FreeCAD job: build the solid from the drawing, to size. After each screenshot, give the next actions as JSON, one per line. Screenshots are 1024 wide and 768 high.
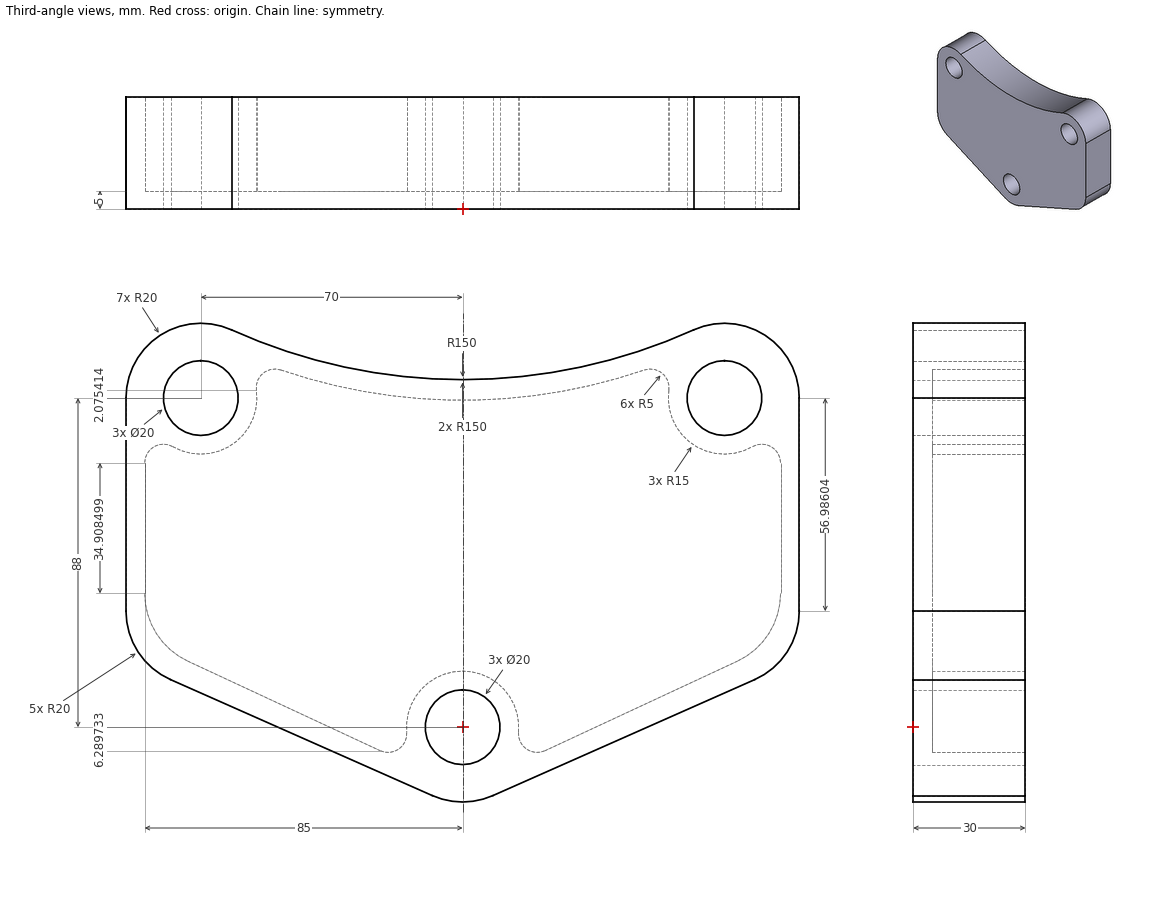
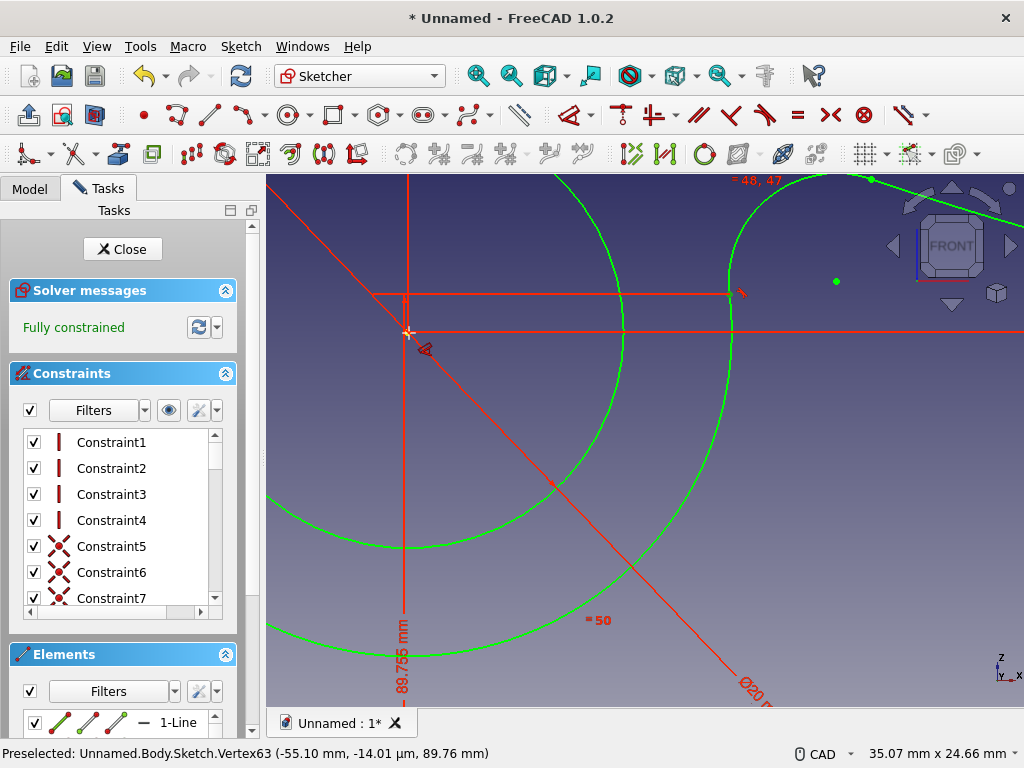
{"action": "left_click", "coordinate": [408, 332]}
{"action": "left_click", "coordinate": [374, 313]}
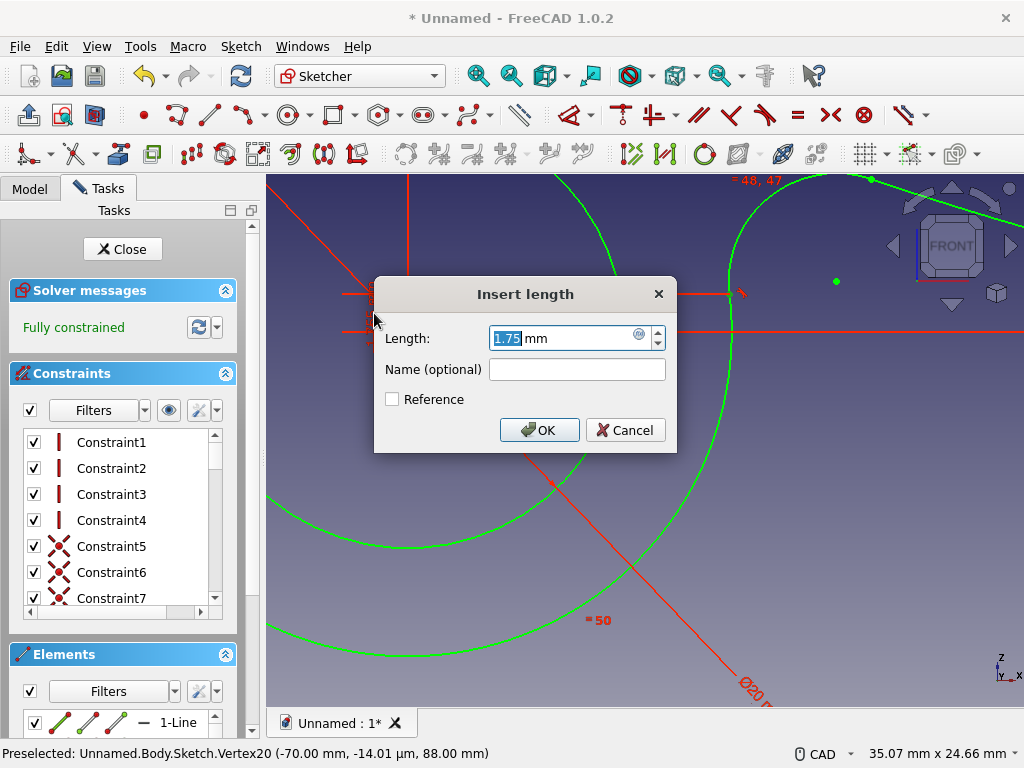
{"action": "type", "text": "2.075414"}
{"action": "key", "text": "Return"}
{"action": "key", "text": "Escape"}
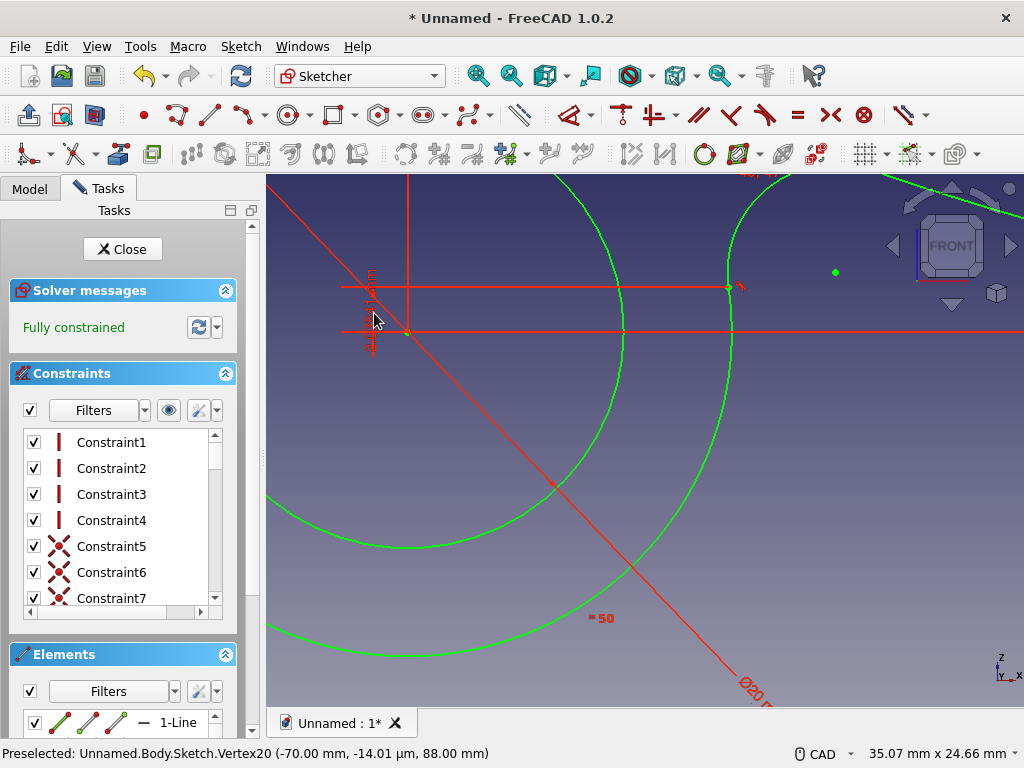
{"action": "left_click", "coordinate": [123, 249]}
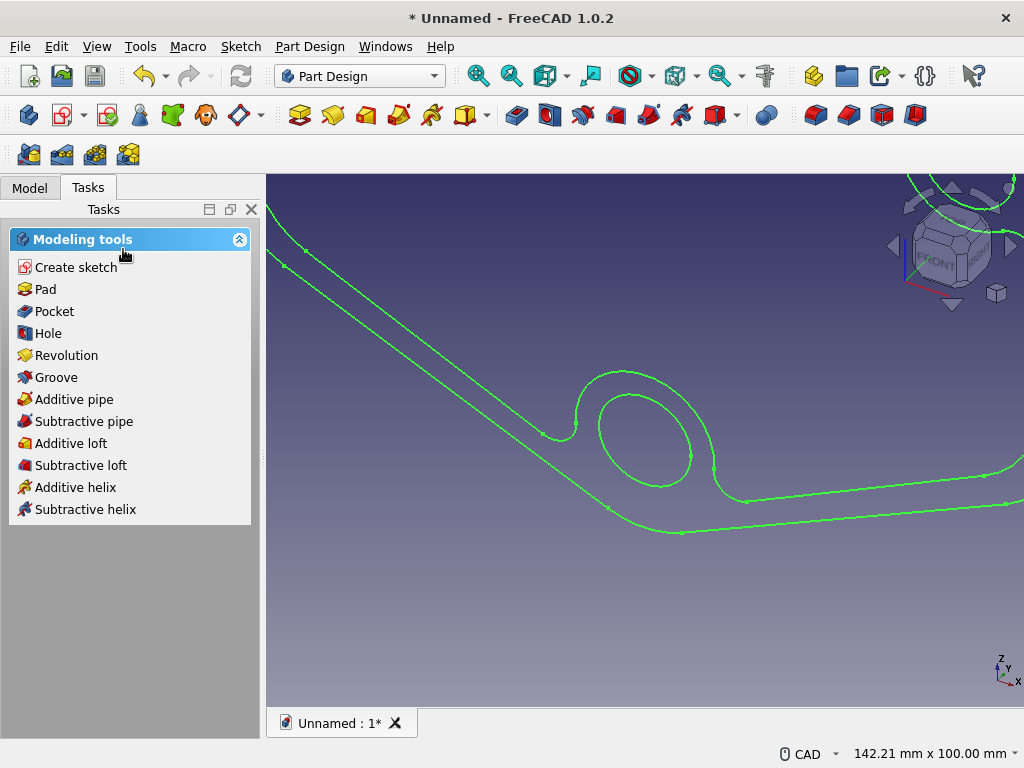
{"action": "left_click", "coordinate": [300, 116]}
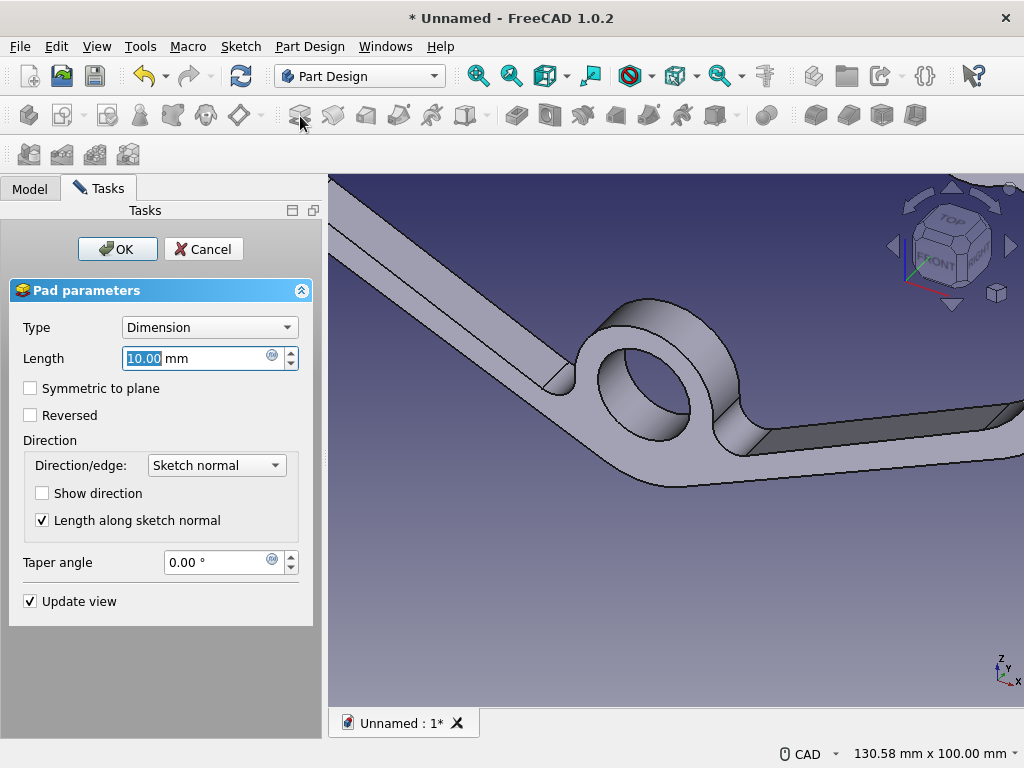
{"action": "type", "text": "30"}
{"action": "key", "text": "Tab"}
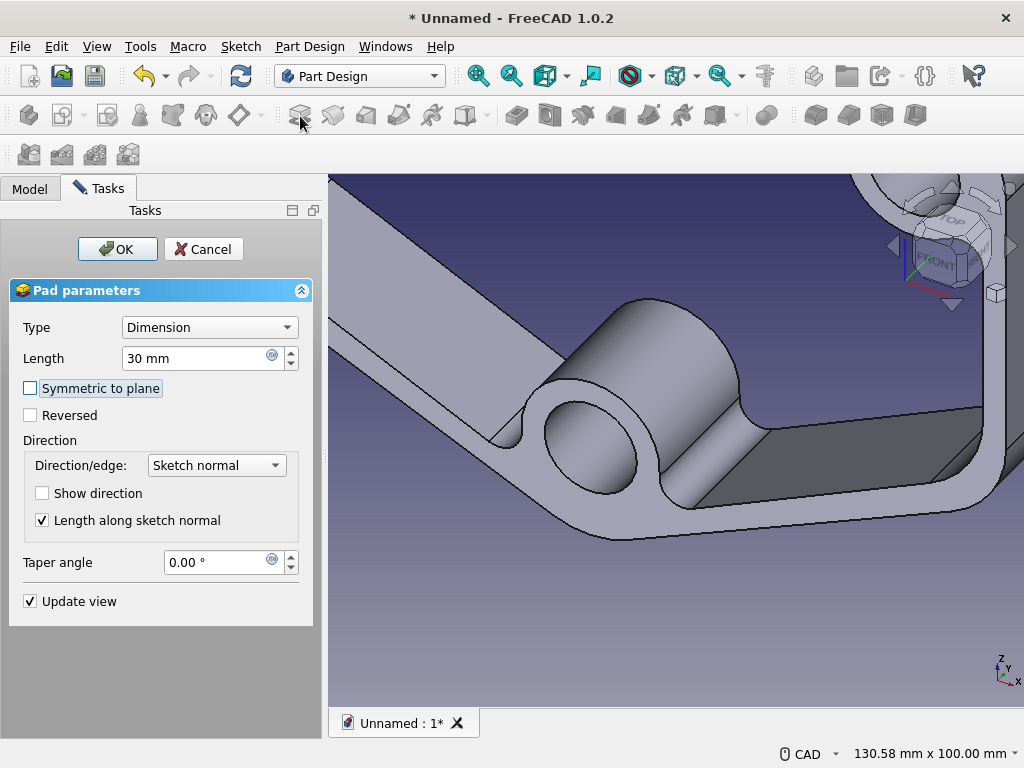
{"action": "left_click", "coordinate": [31, 415]}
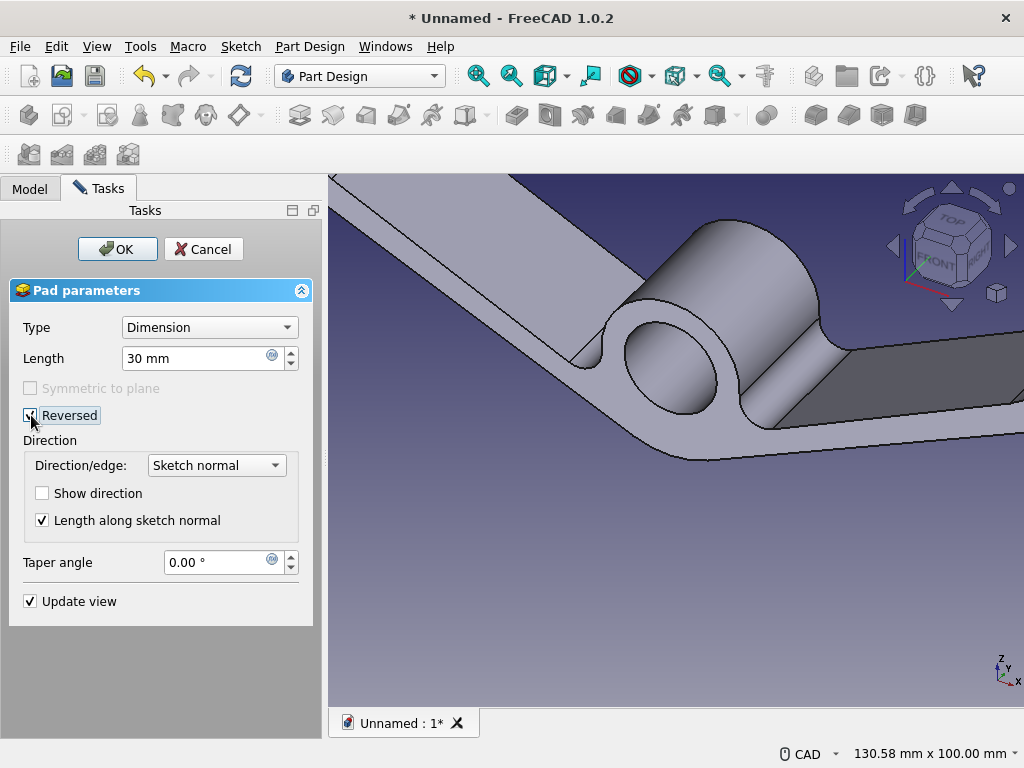
{"action": "left_click", "coordinate": [118, 249]}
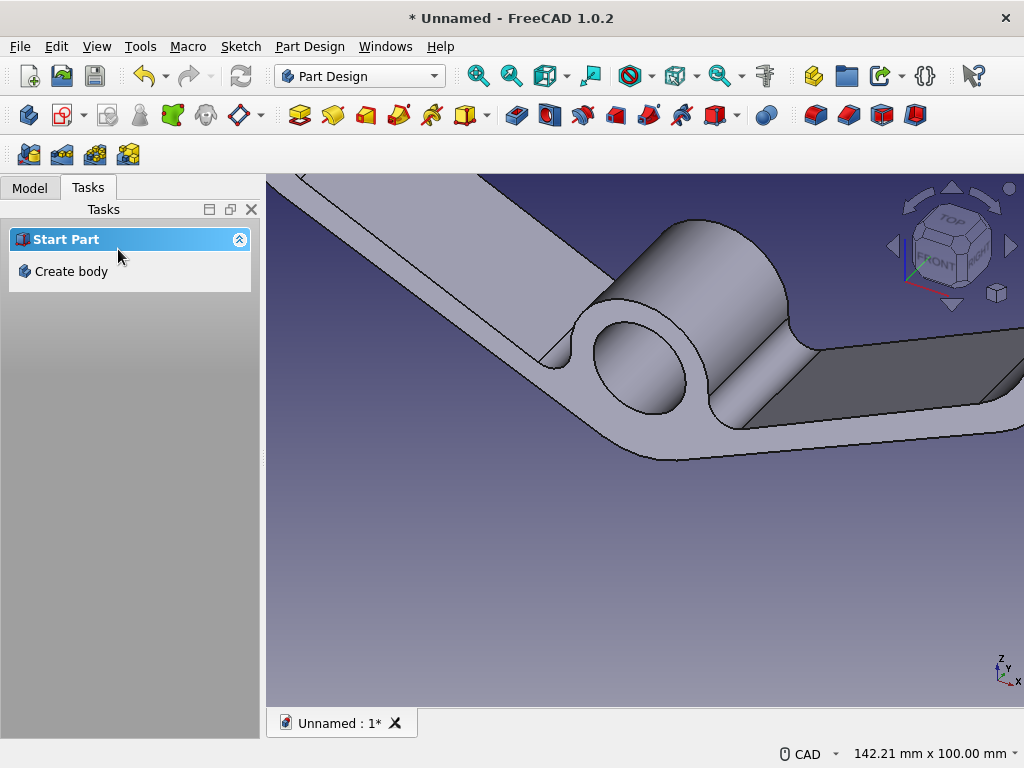
{"action": "left_click", "coordinate": [479, 76]}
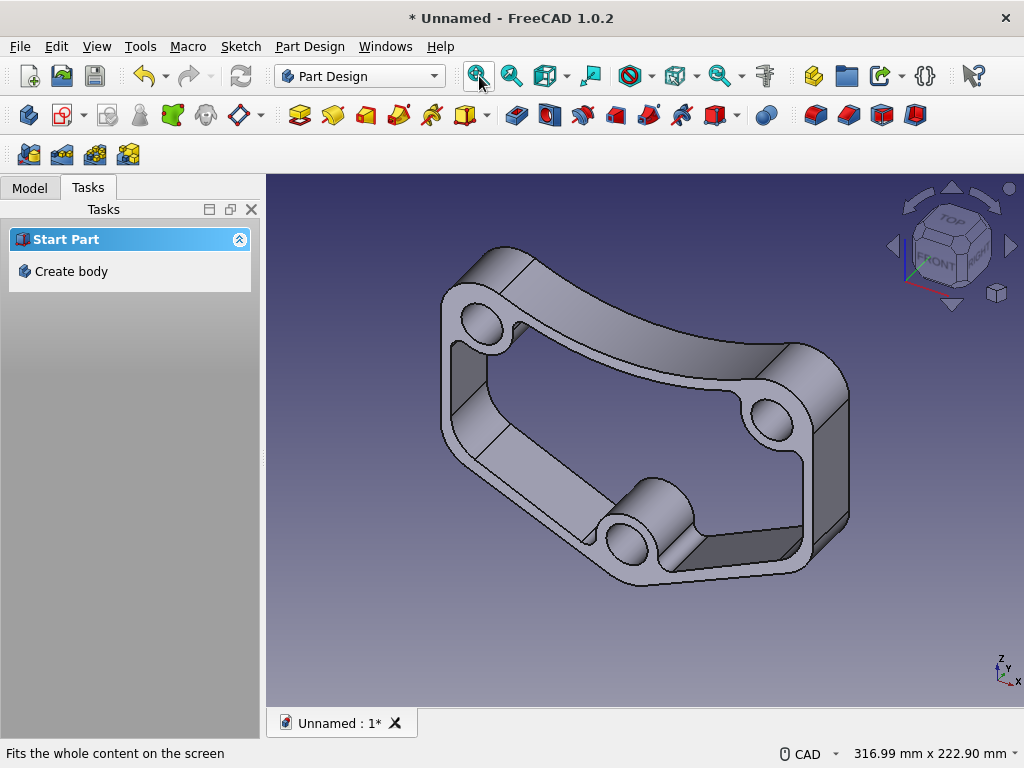
{"action": "left_click", "coordinate": [787, 403]}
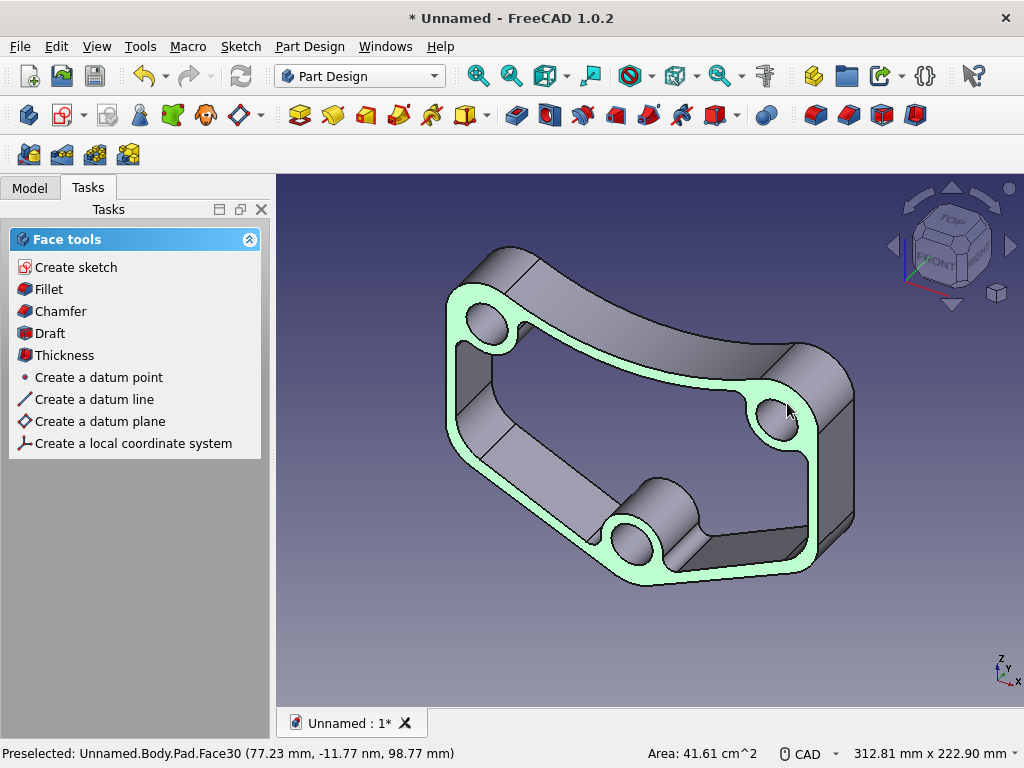
{"action": "left_click", "coordinate": [62, 116]}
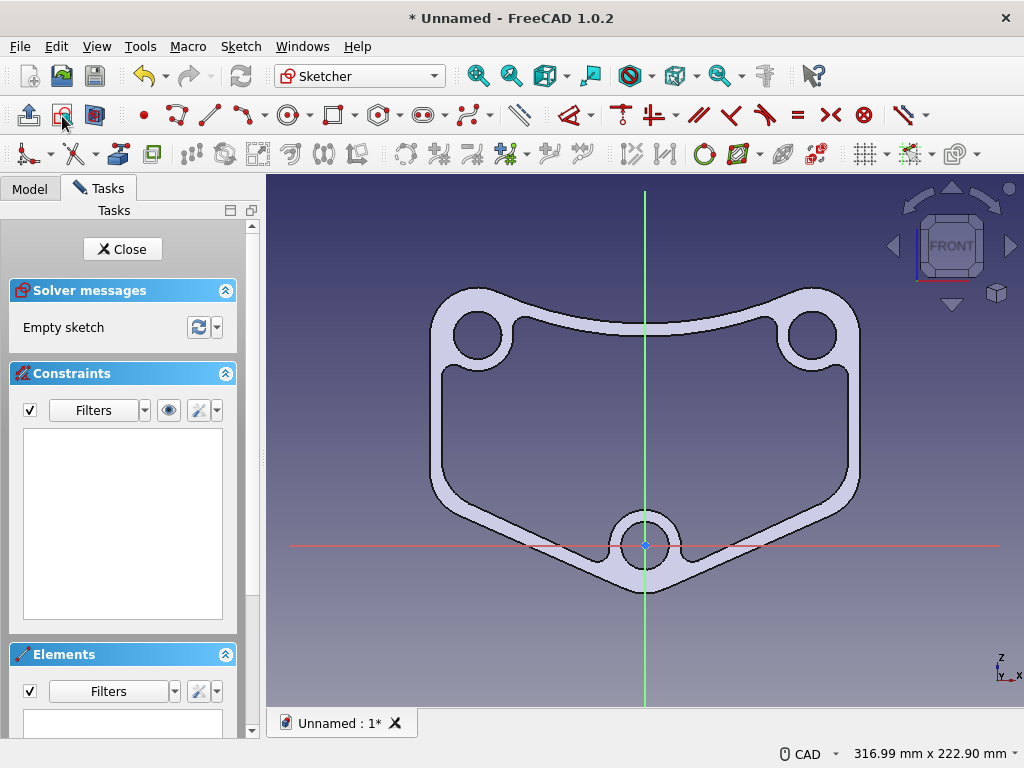
{"action": "scroll", "coordinate": [294, 431], "scroll_direction": "down", "scroll_amount": 1}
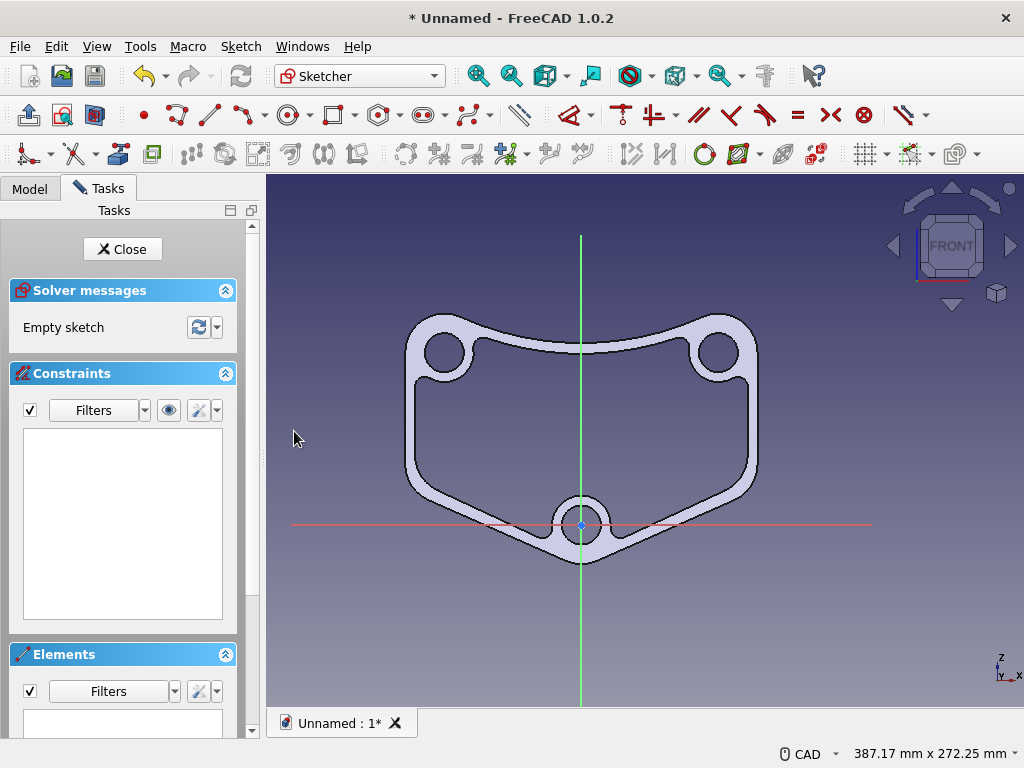
{"action": "left_click", "coordinate": [210, 116]}